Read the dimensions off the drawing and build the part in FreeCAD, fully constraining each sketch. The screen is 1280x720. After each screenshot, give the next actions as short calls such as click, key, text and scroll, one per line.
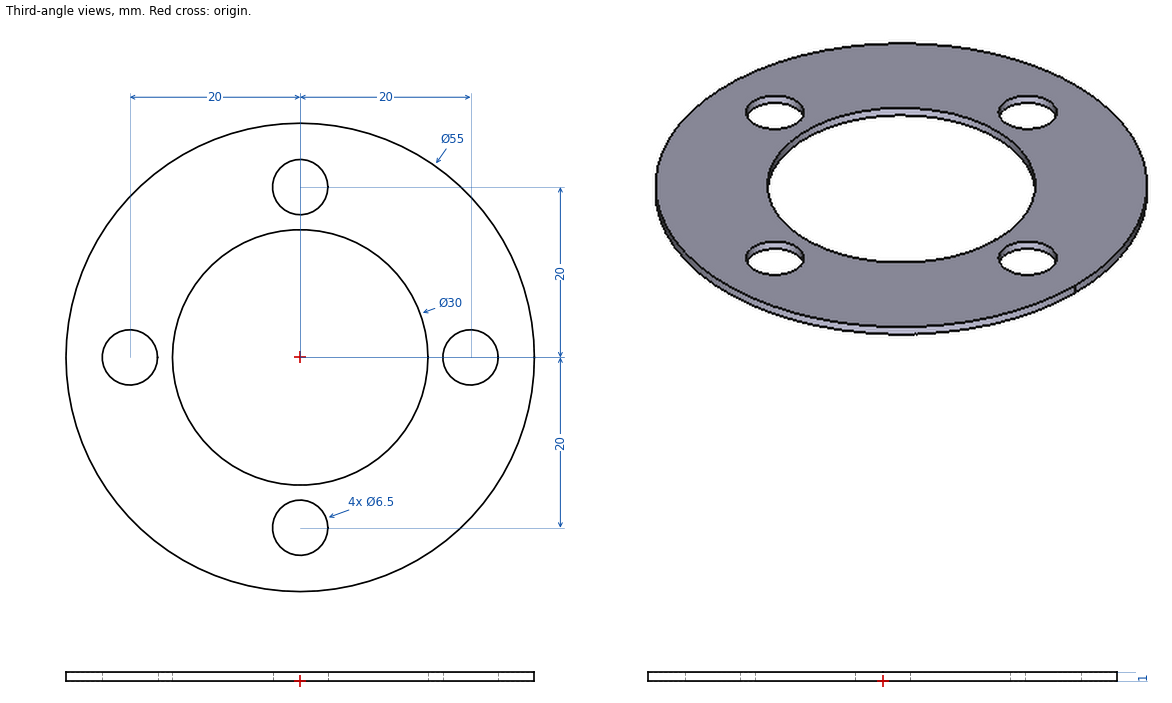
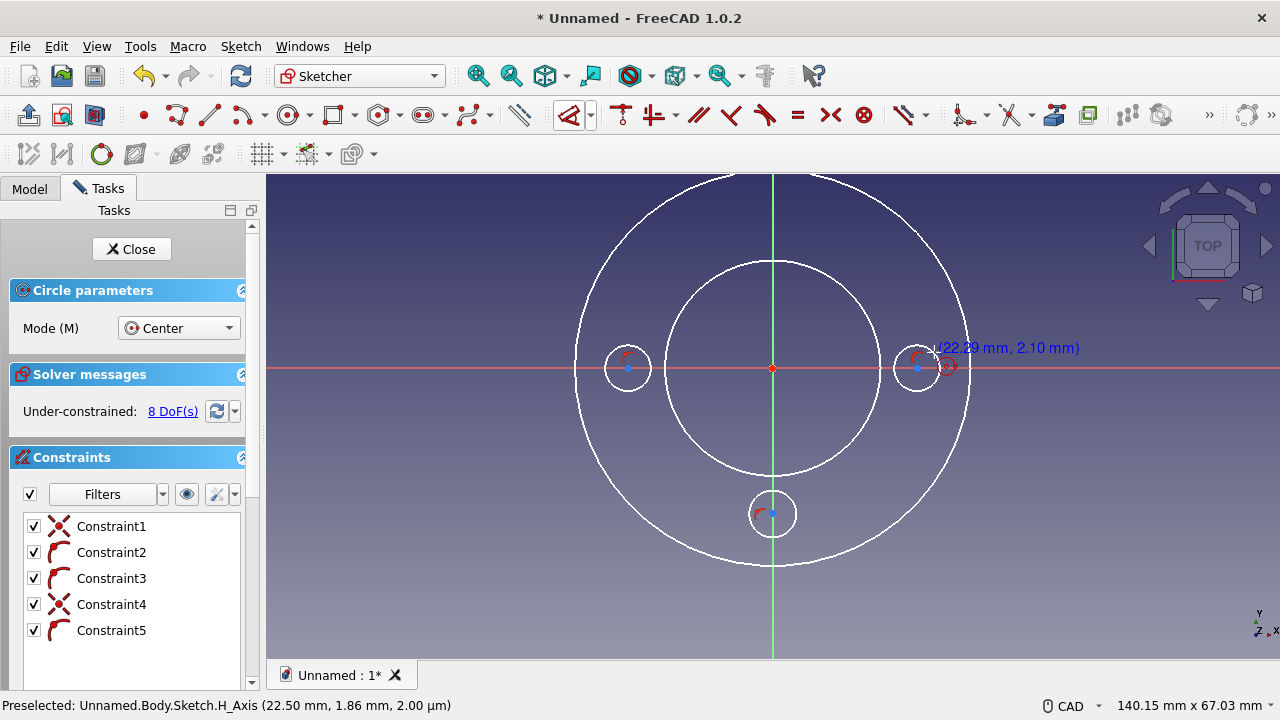
click(773, 223)
click(789, 207)
key(Escape)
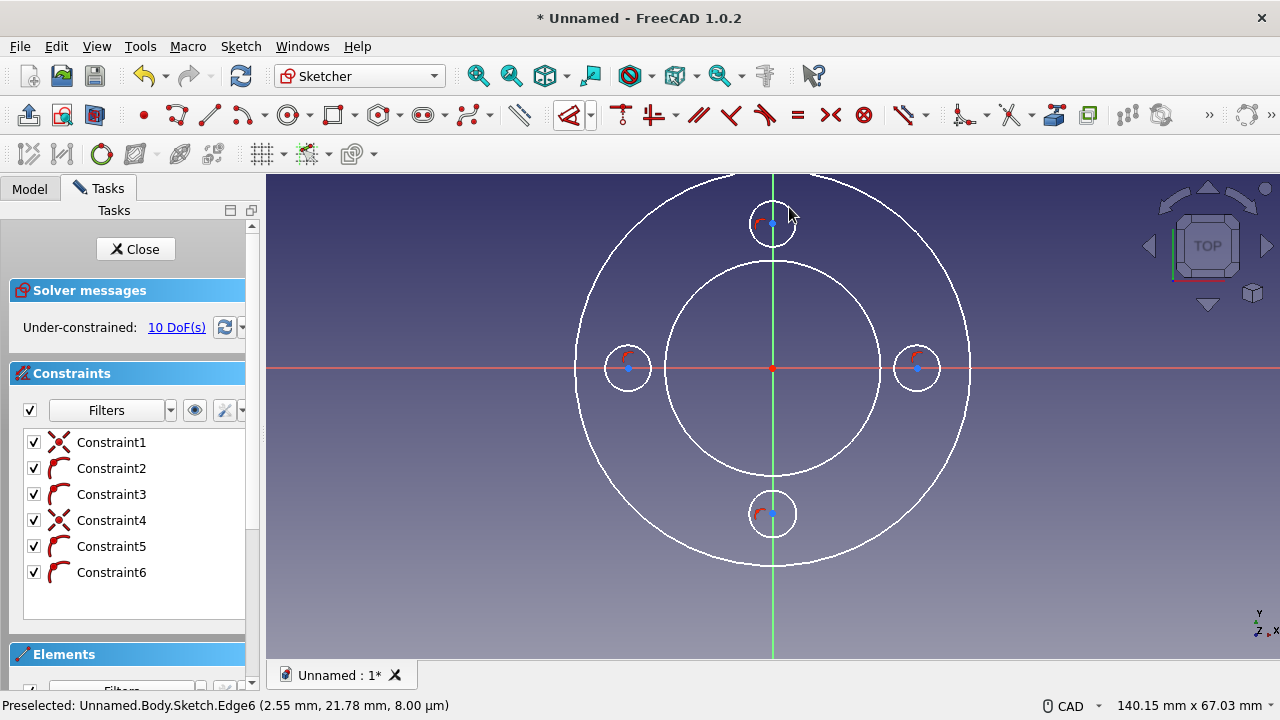
click(789, 497)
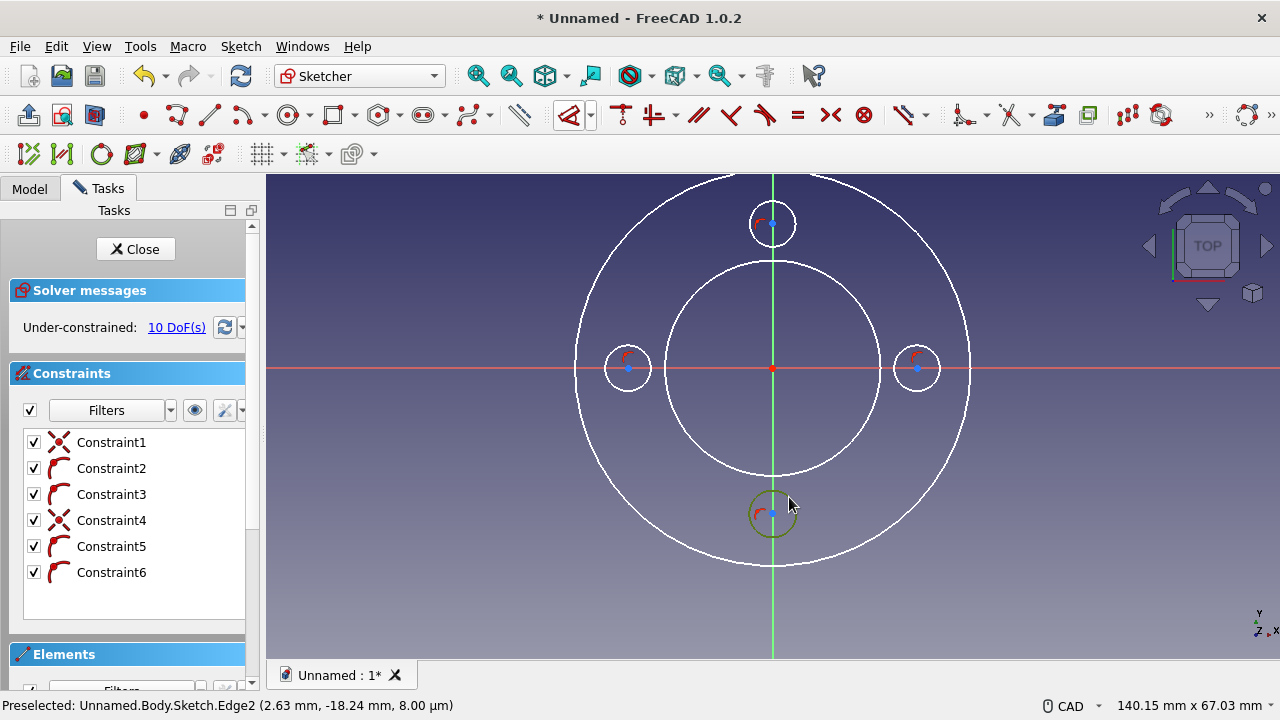
click(644, 352)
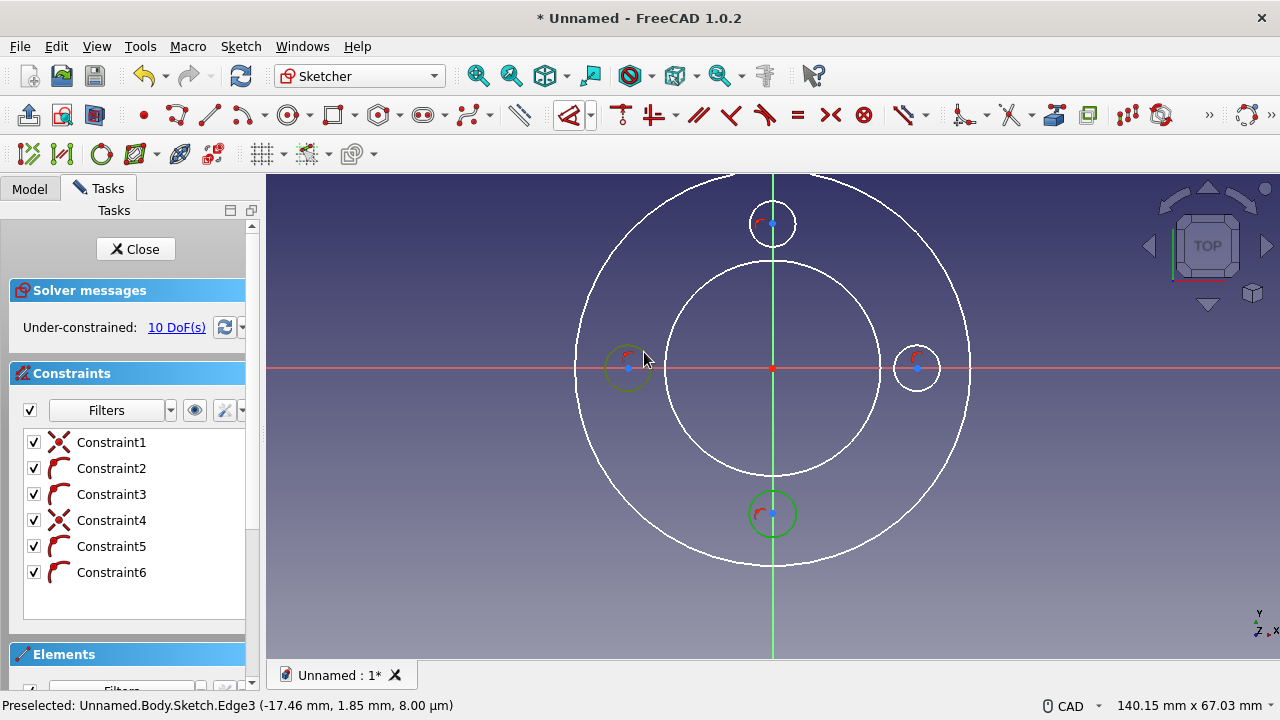
click(933, 352)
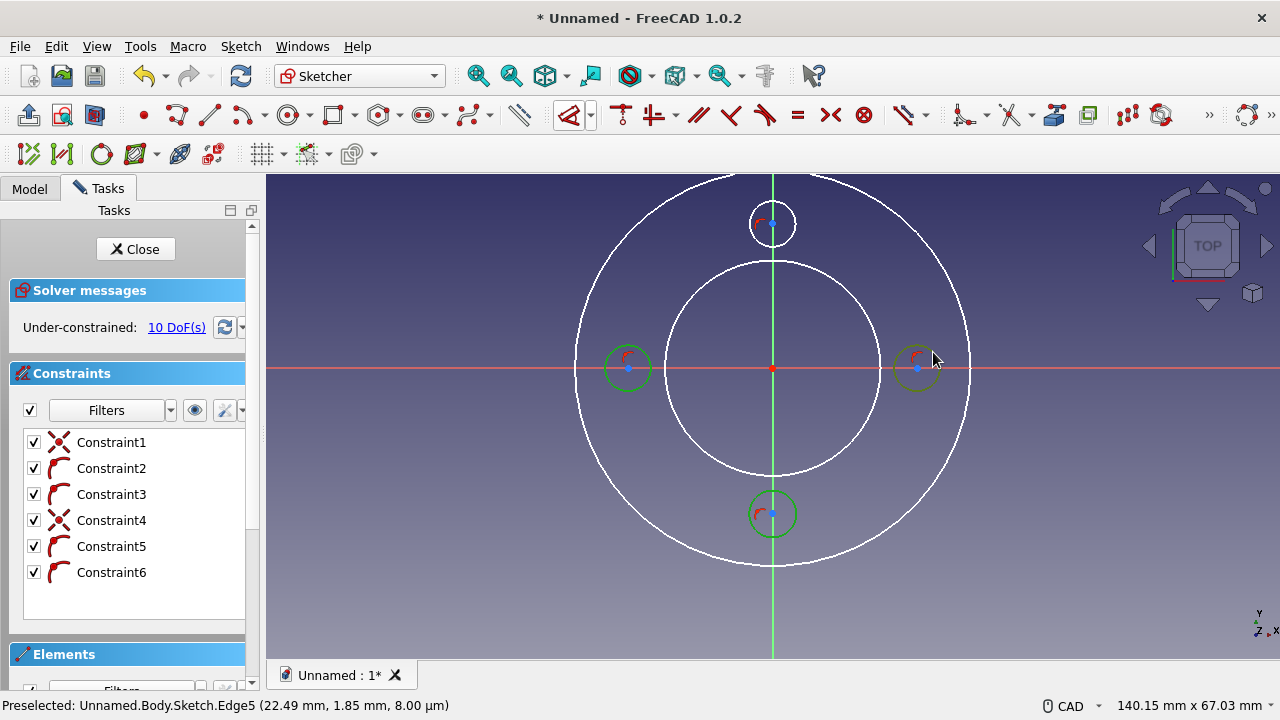
click(789, 208)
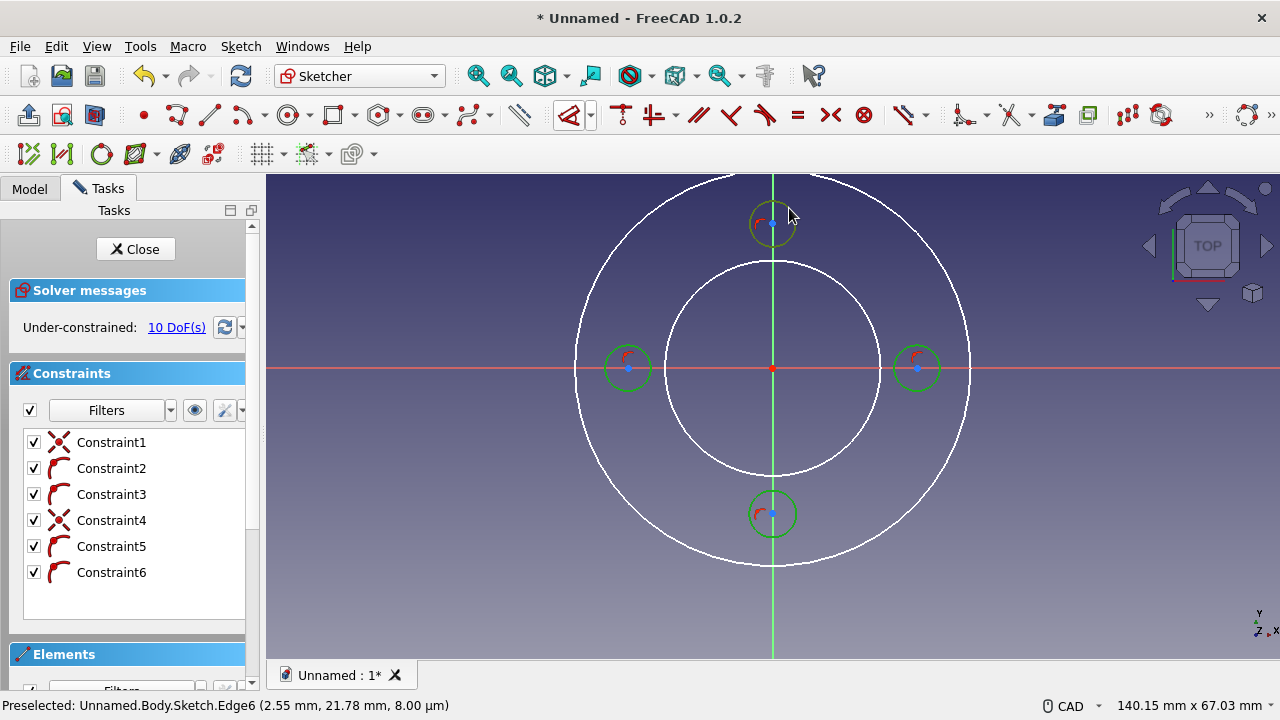
key(e)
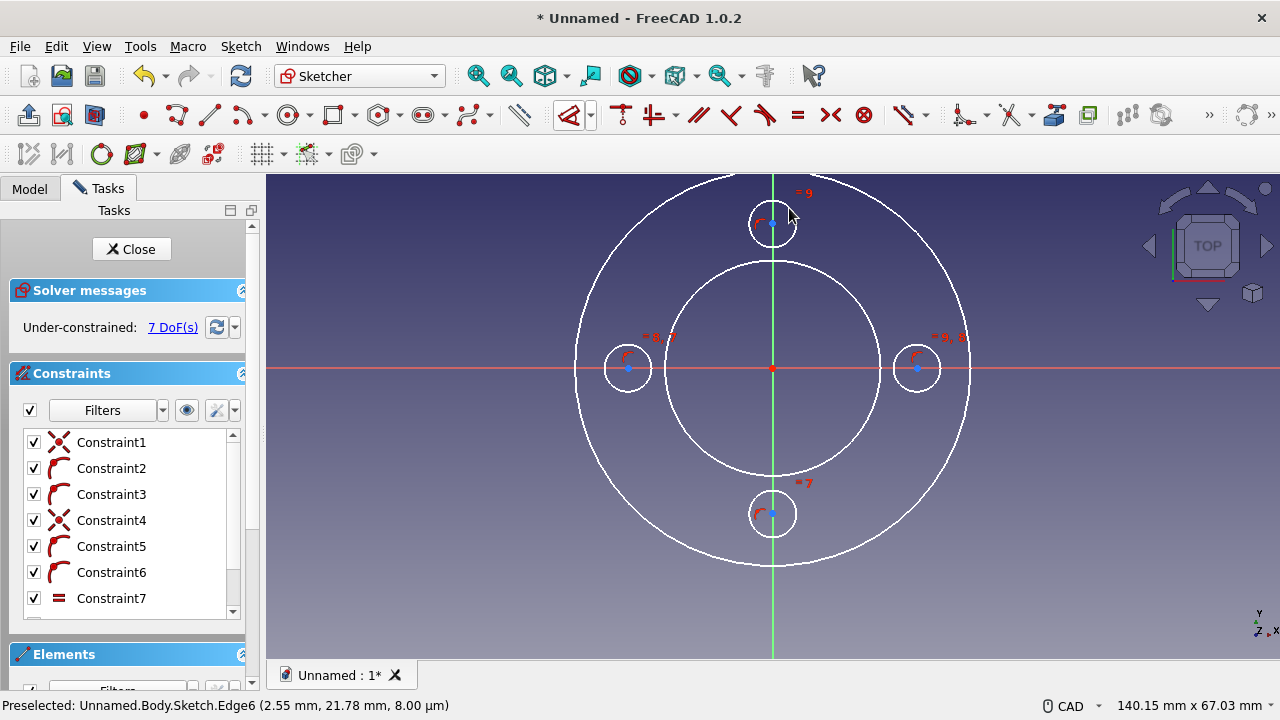
click(568, 116)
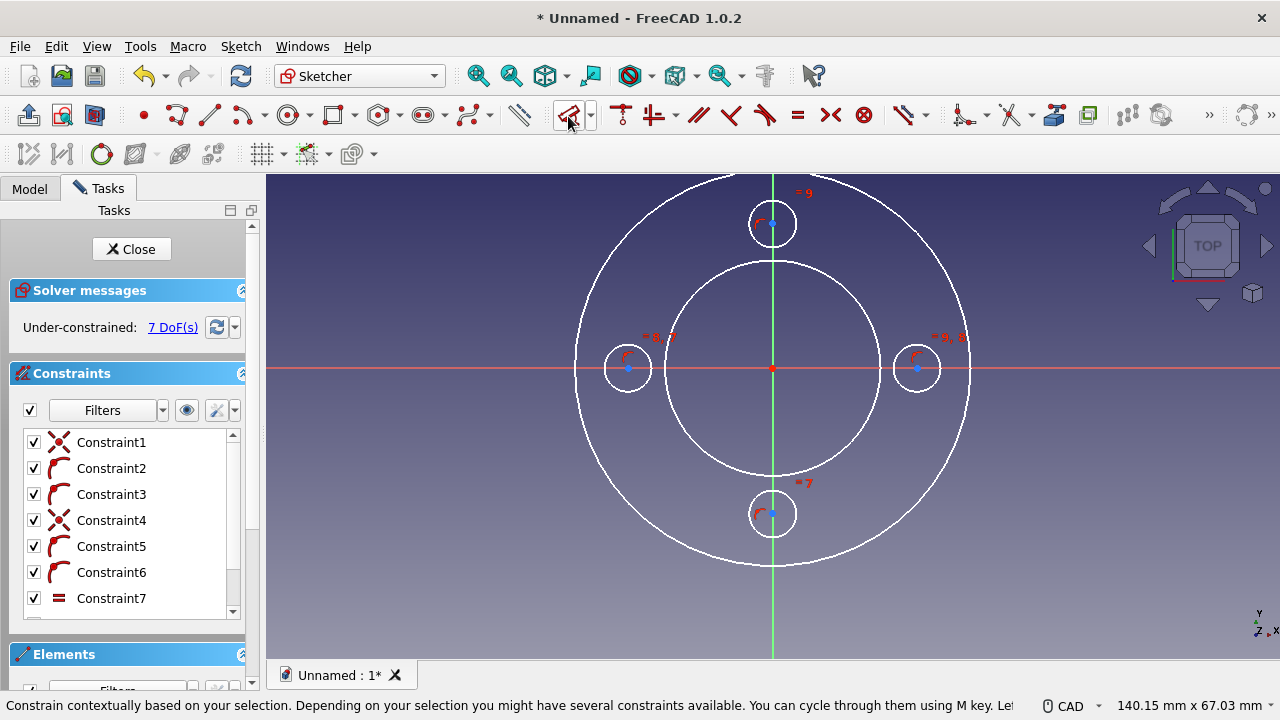
click(912, 228)
click(935, 205)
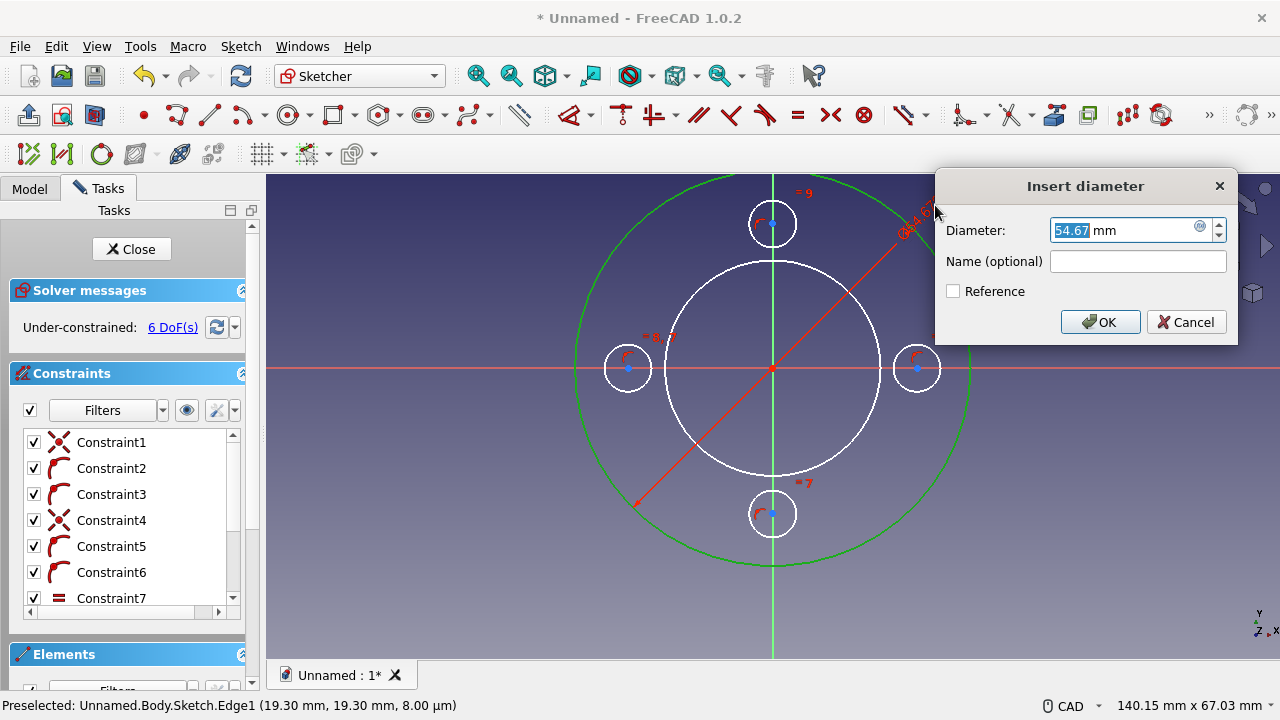
text(55)
key(Return)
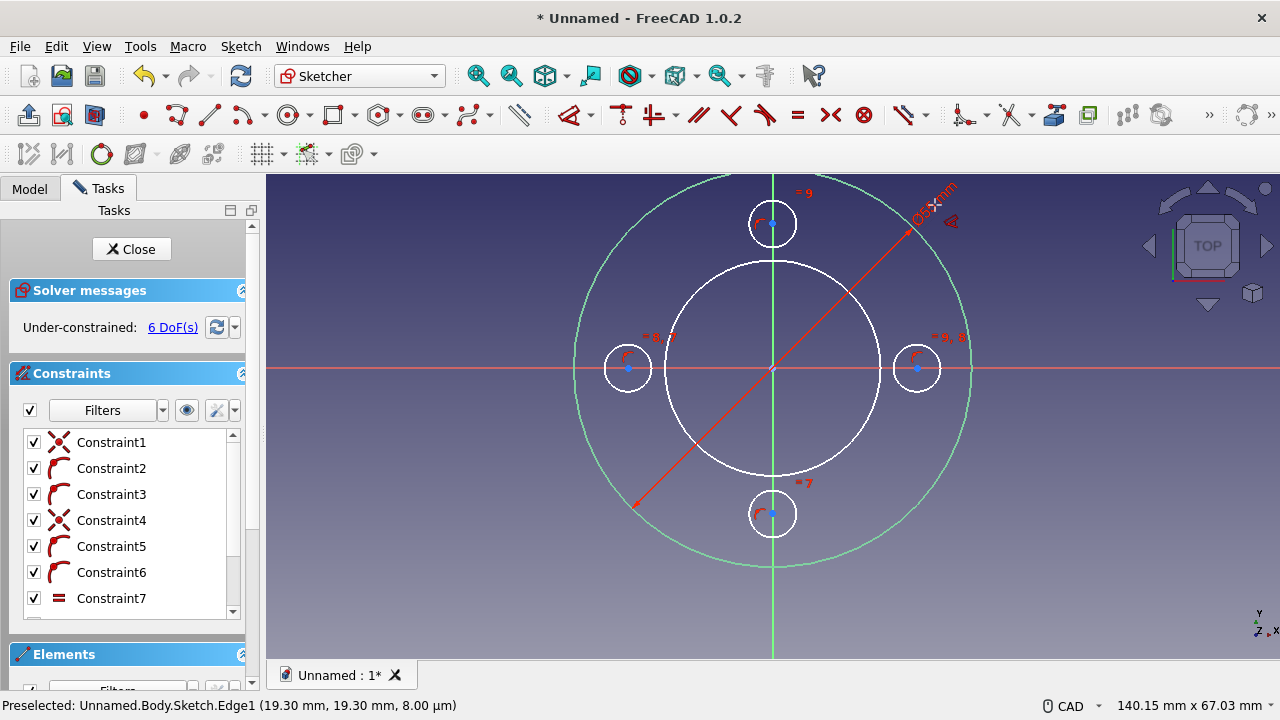
click(789, 497)
click(826, 497)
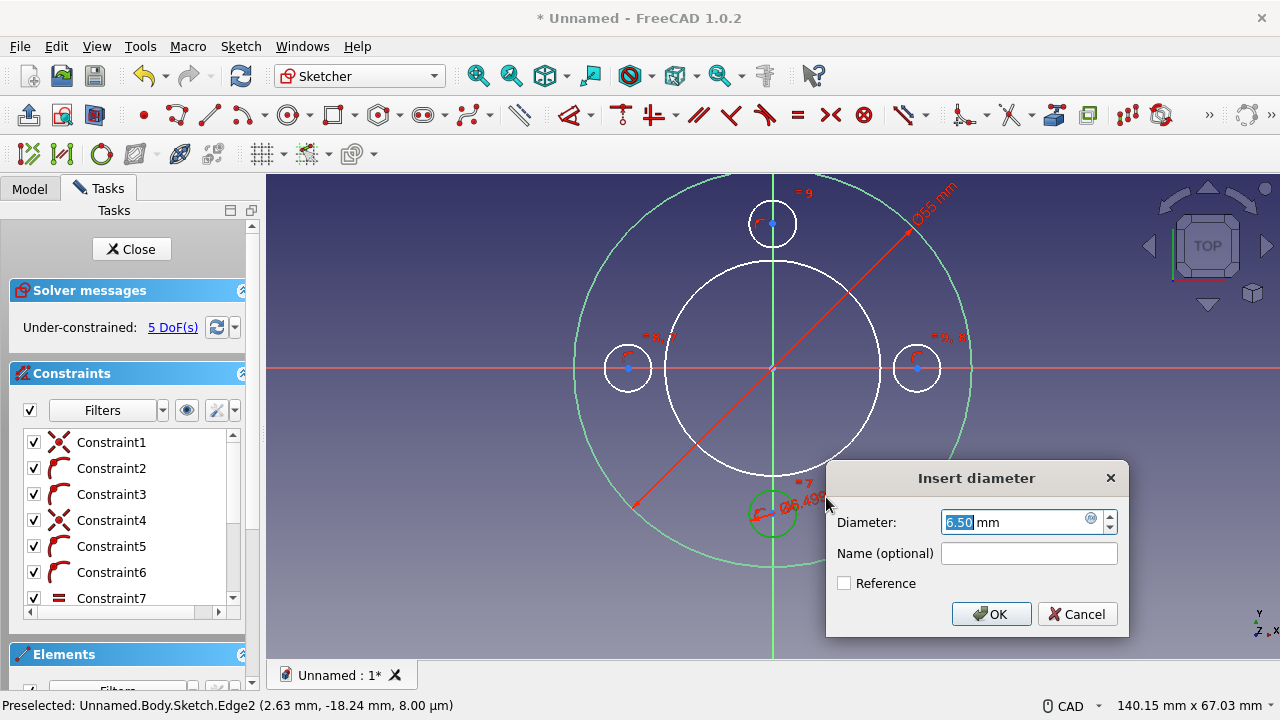
text(6.5)
key(Return)